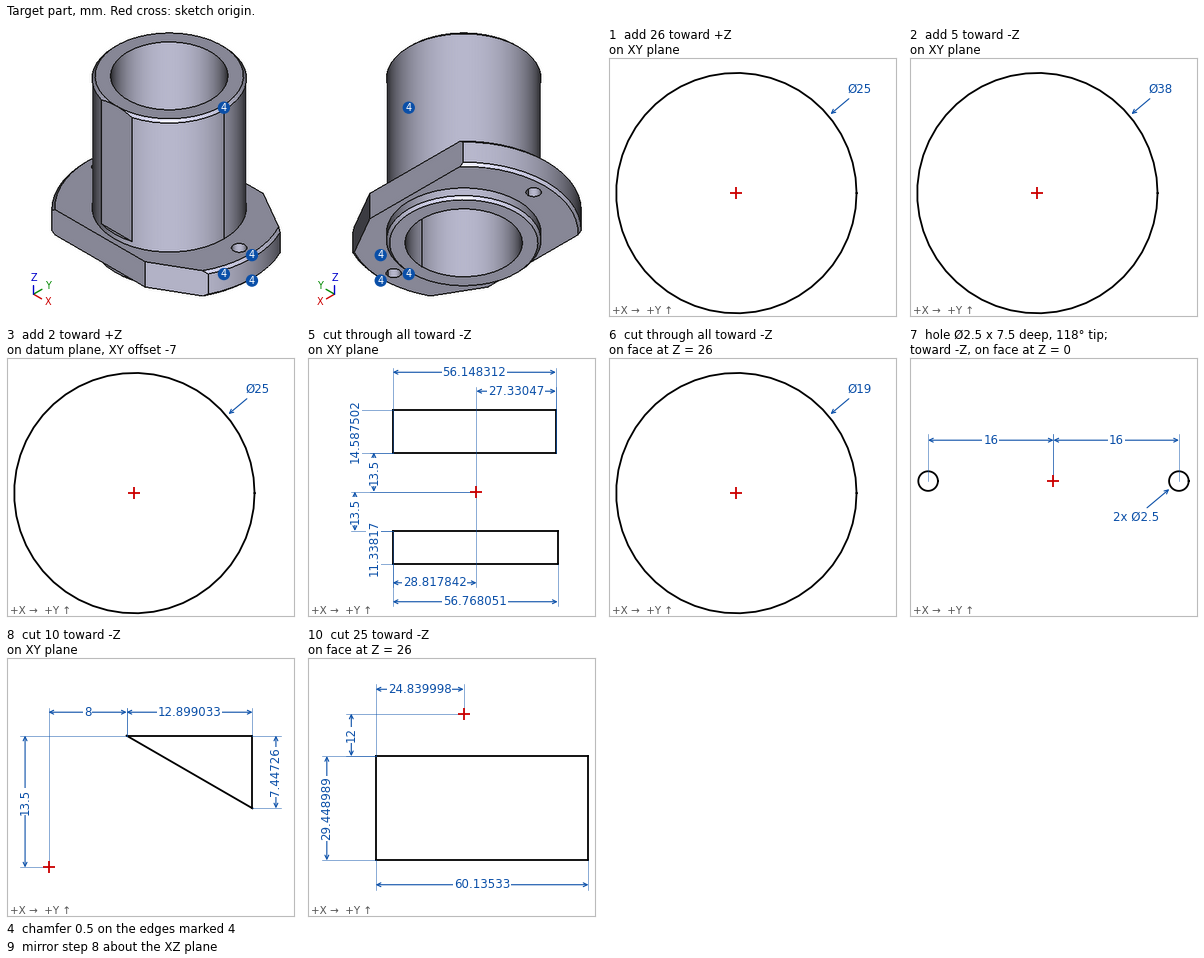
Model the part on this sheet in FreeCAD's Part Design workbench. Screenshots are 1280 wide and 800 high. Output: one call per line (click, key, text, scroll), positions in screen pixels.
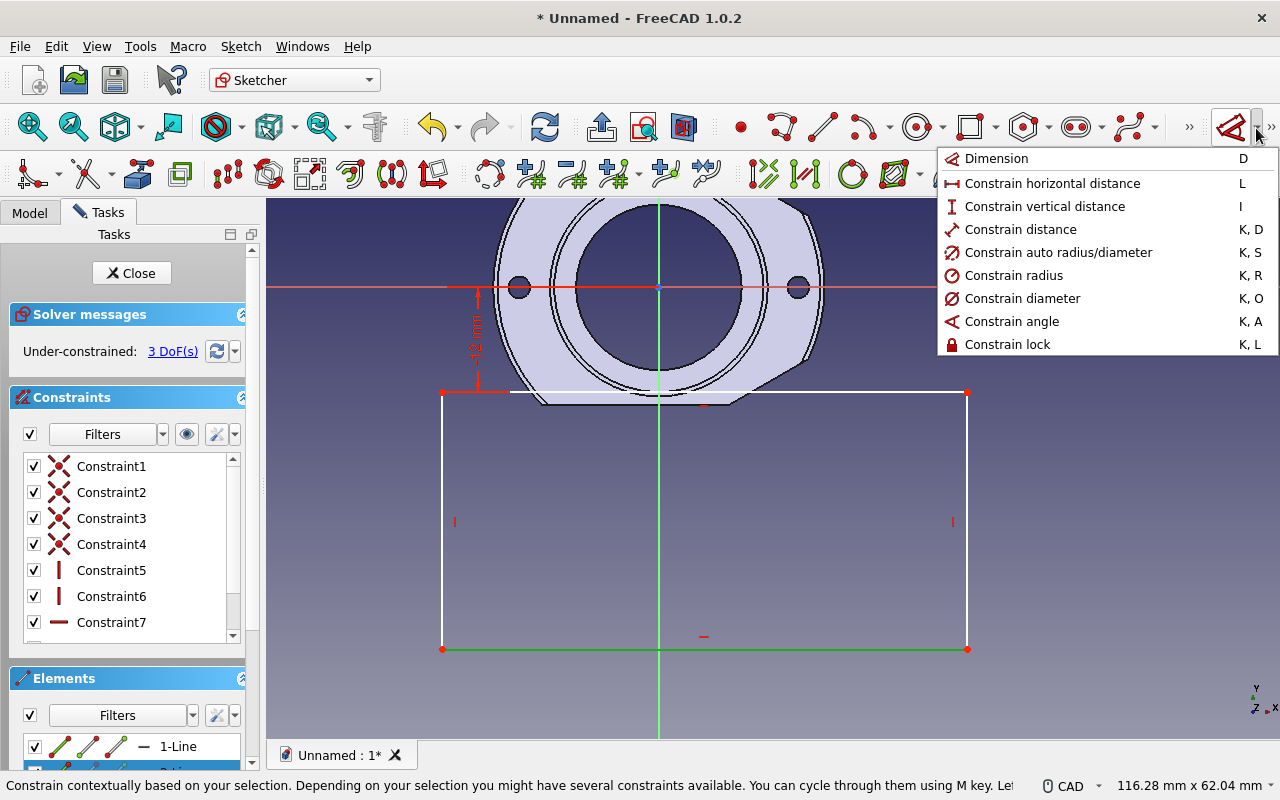
click(1108, 184)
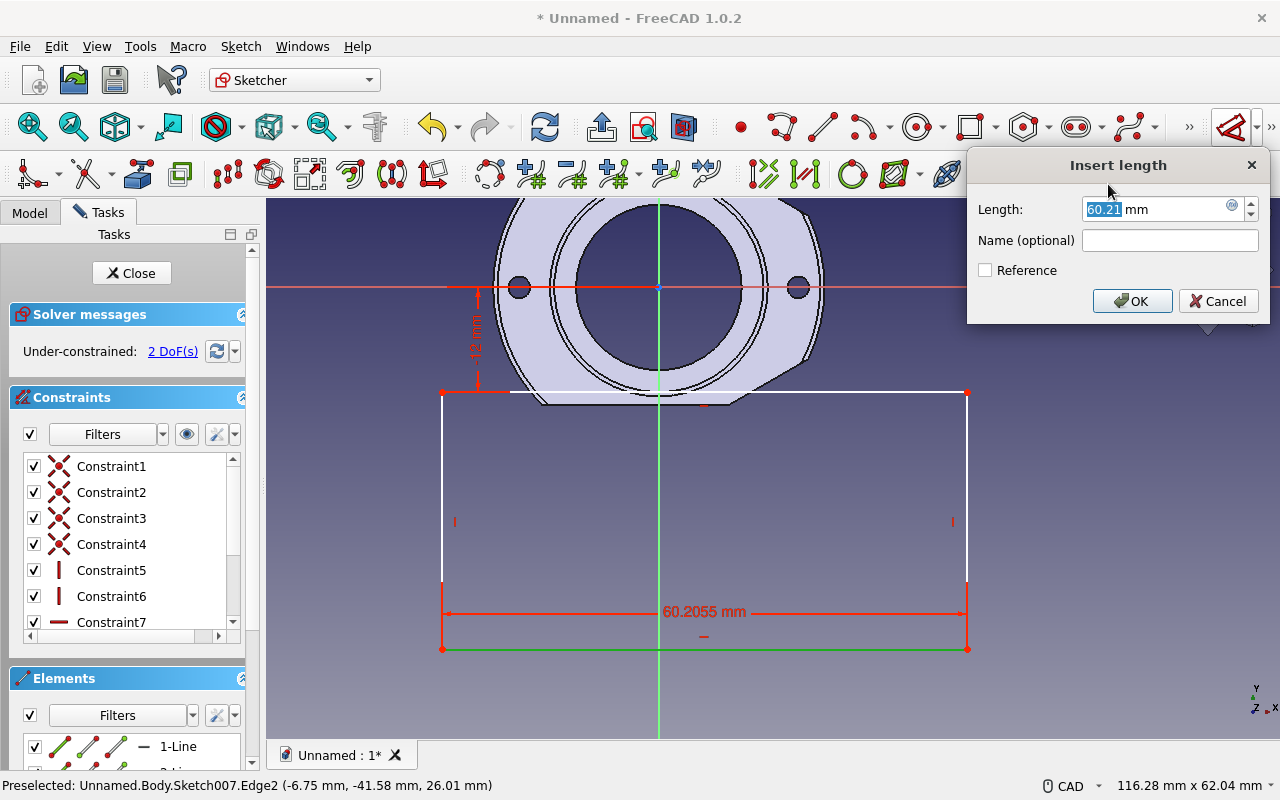
text(60.13533)
key(Return)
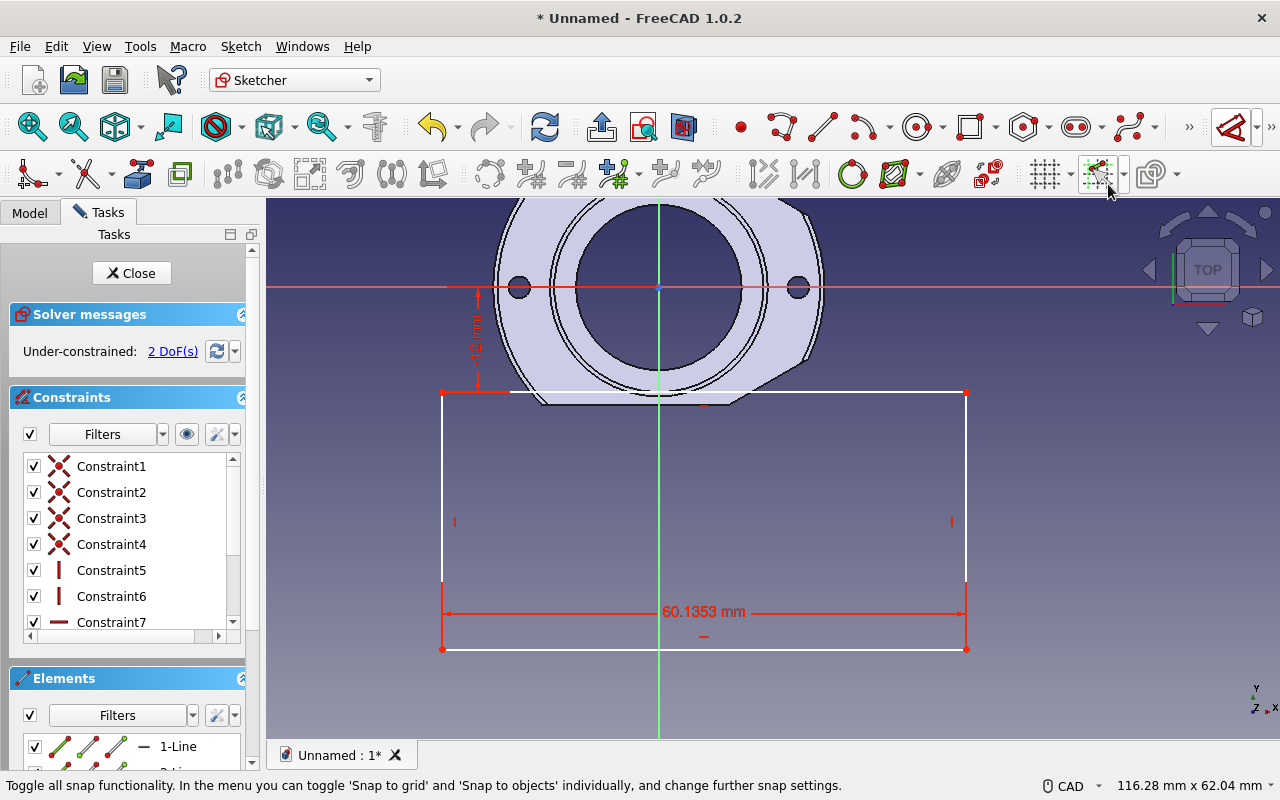
click(442, 469)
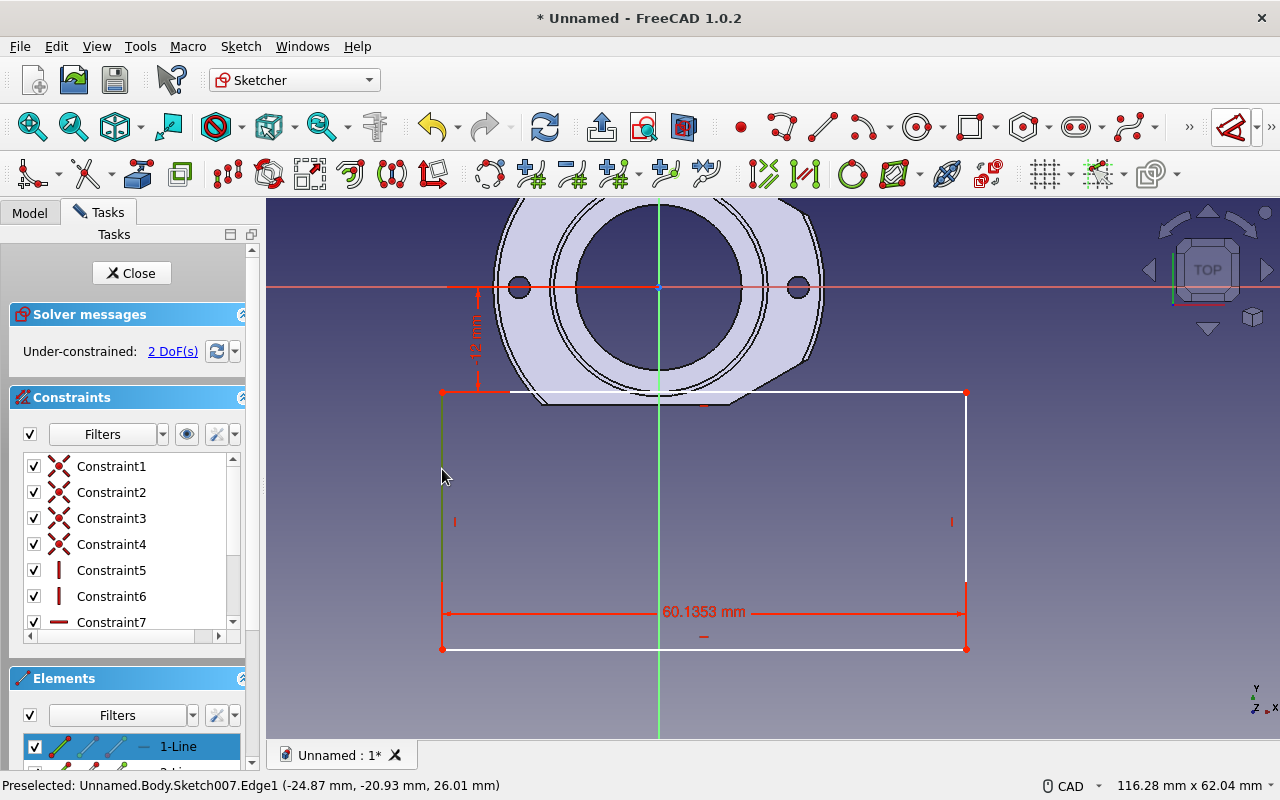
key(i)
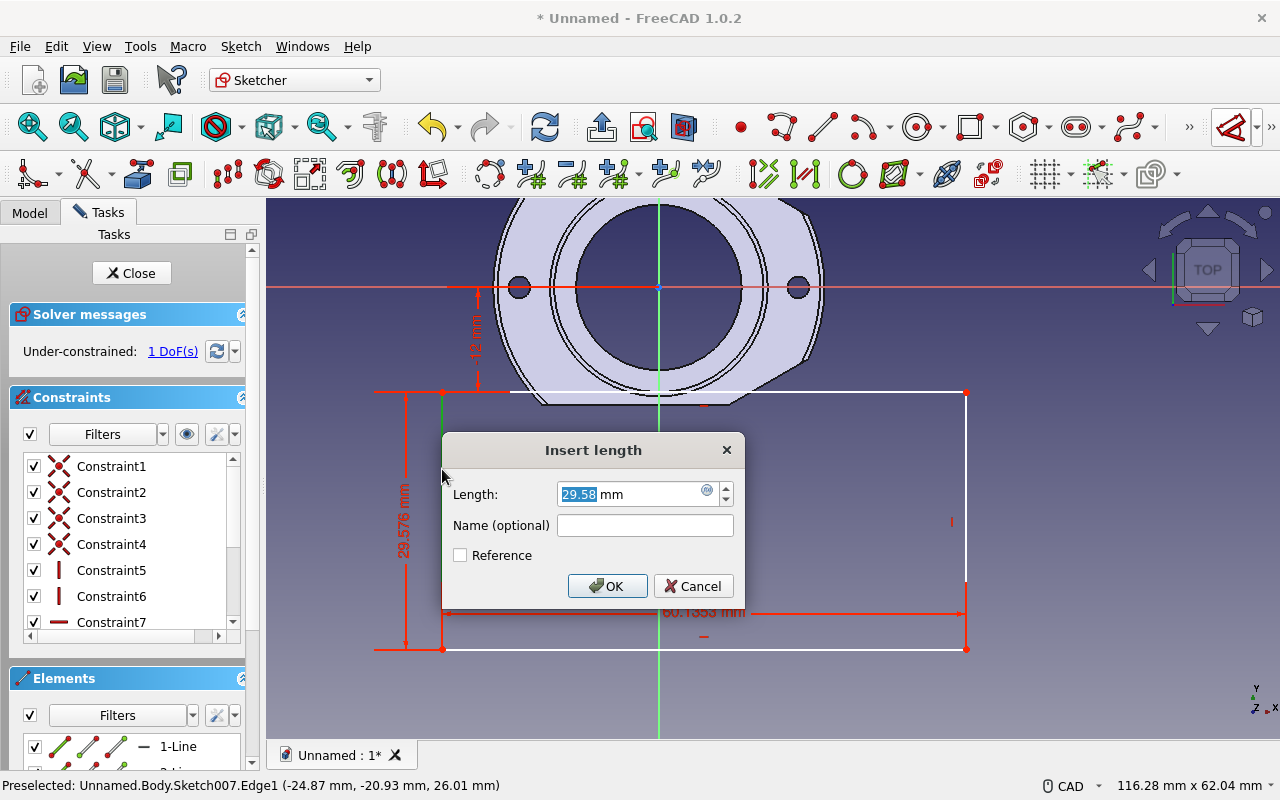
text(29.448989)
key(Return)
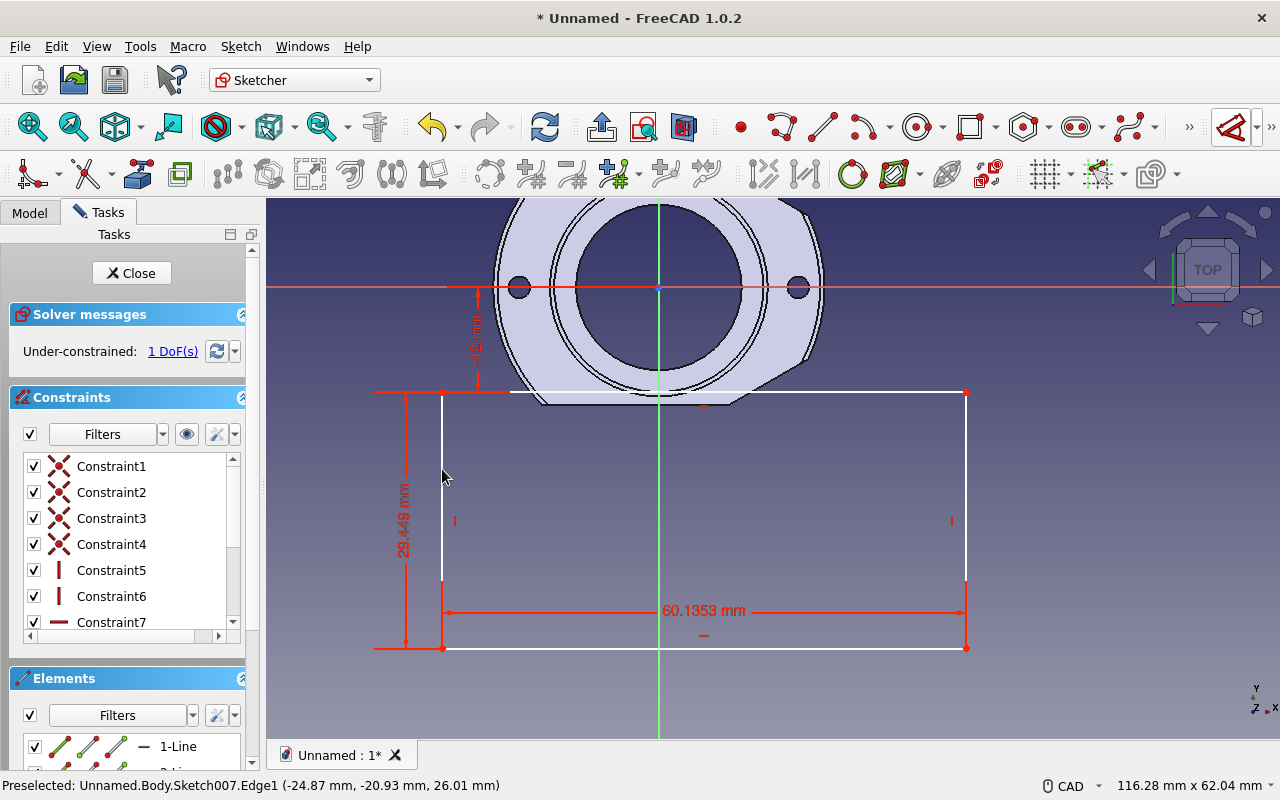
click(442, 392)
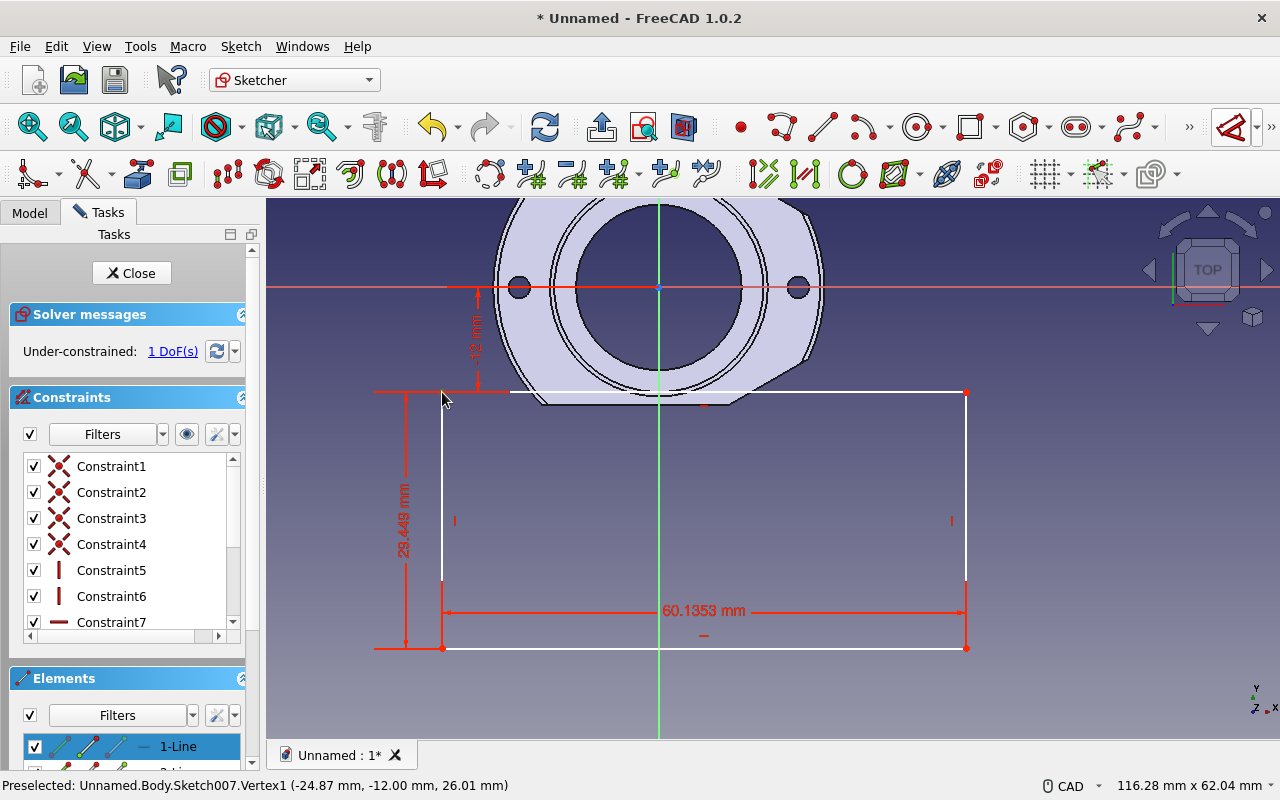
key(l)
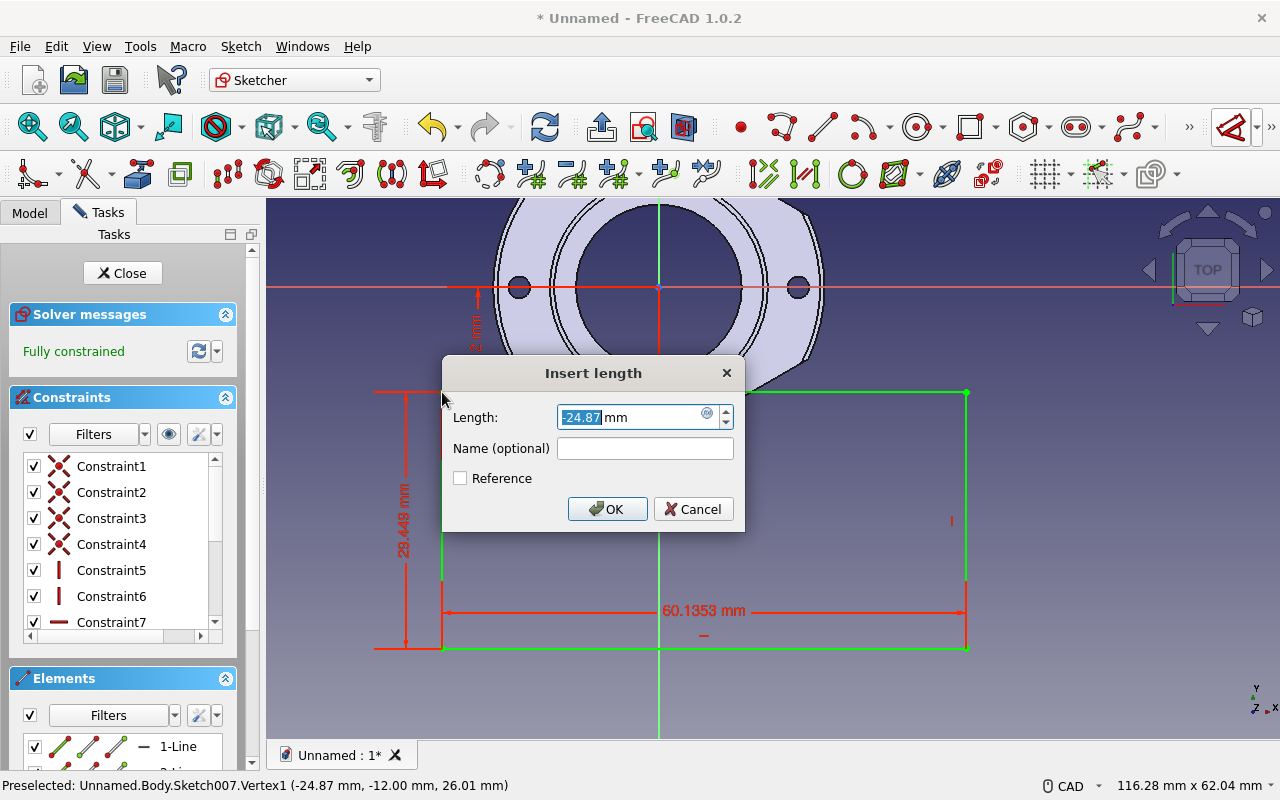
text(-24.839998)
key(Return)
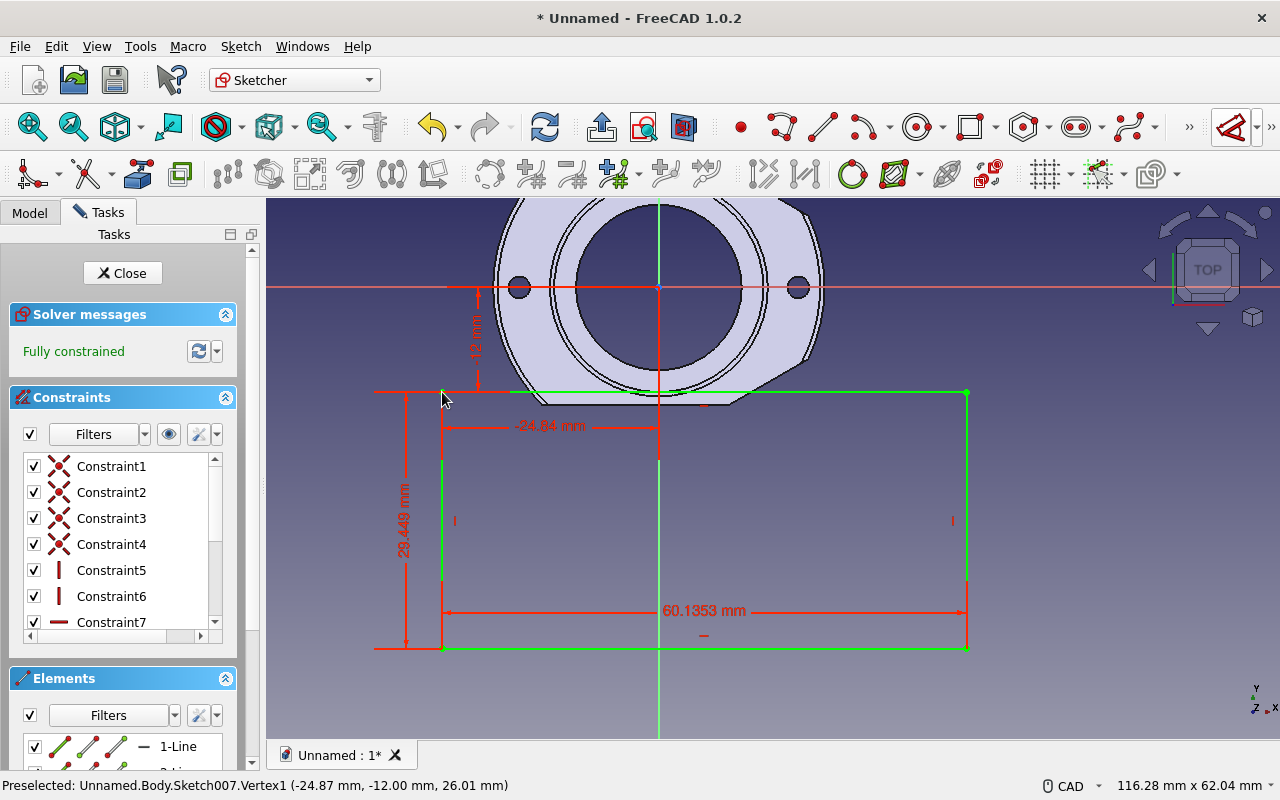
click(123, 273)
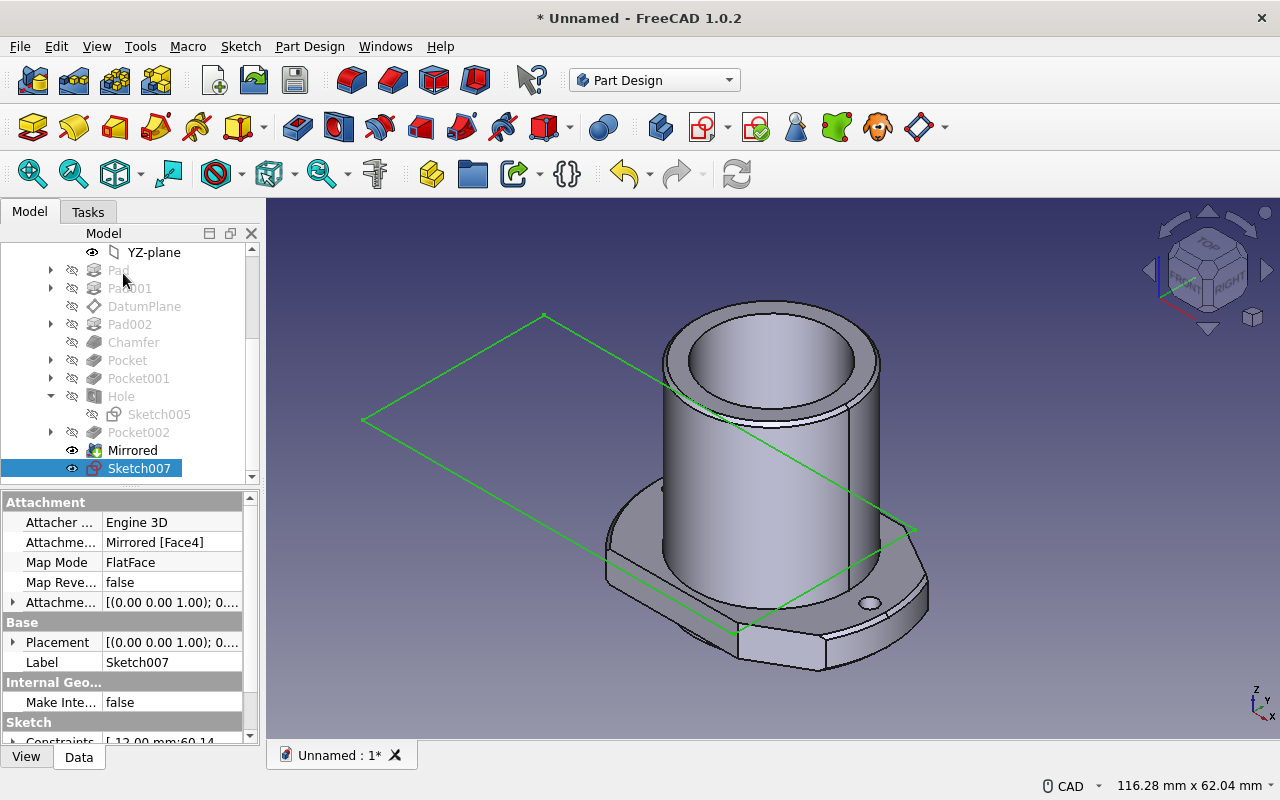
click(298, 128)